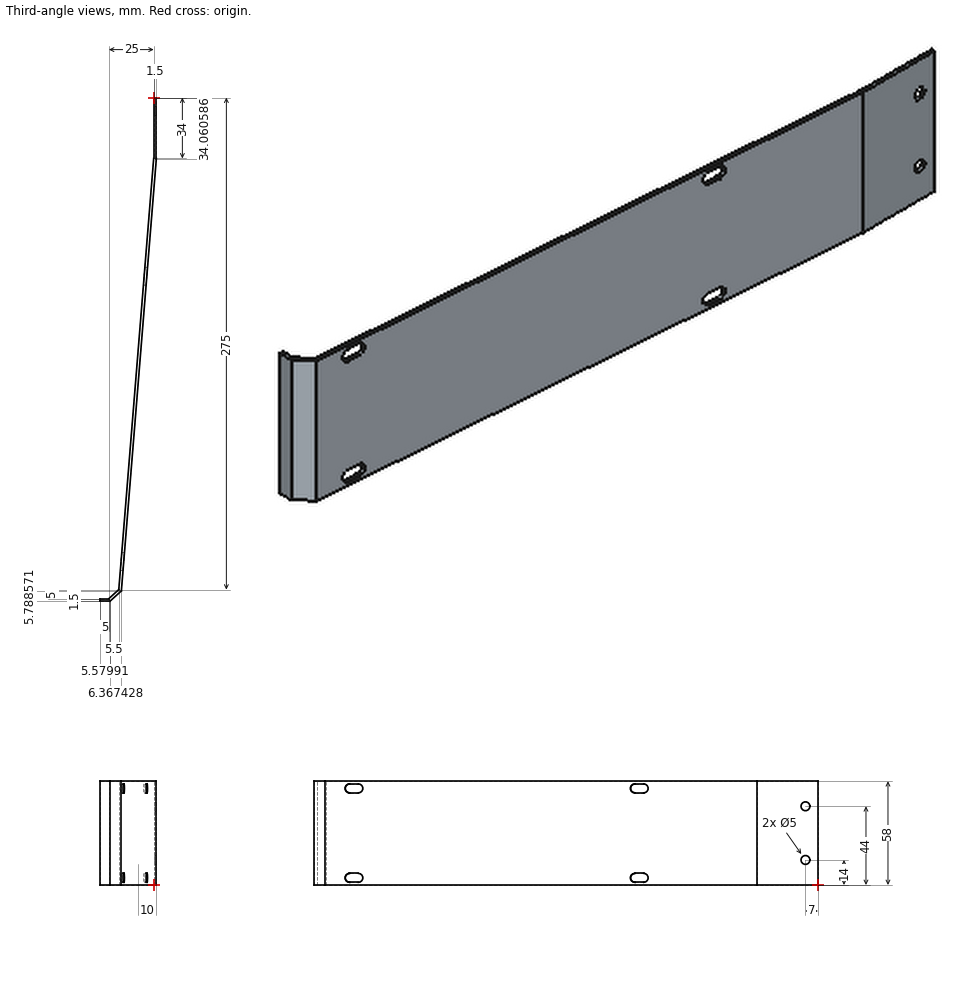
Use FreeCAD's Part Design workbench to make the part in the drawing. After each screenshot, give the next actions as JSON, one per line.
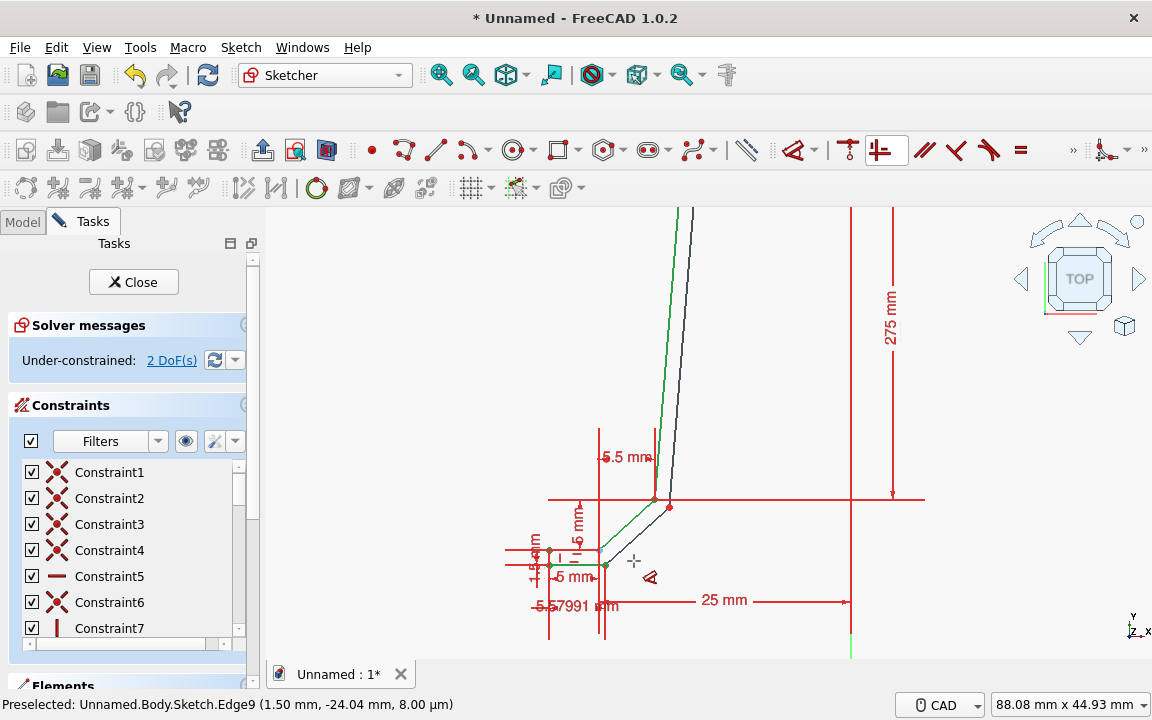
{"action": "left_click", "coordinate": [624, 548]}
{"action": "left_click", "coordinate": [652, 599]}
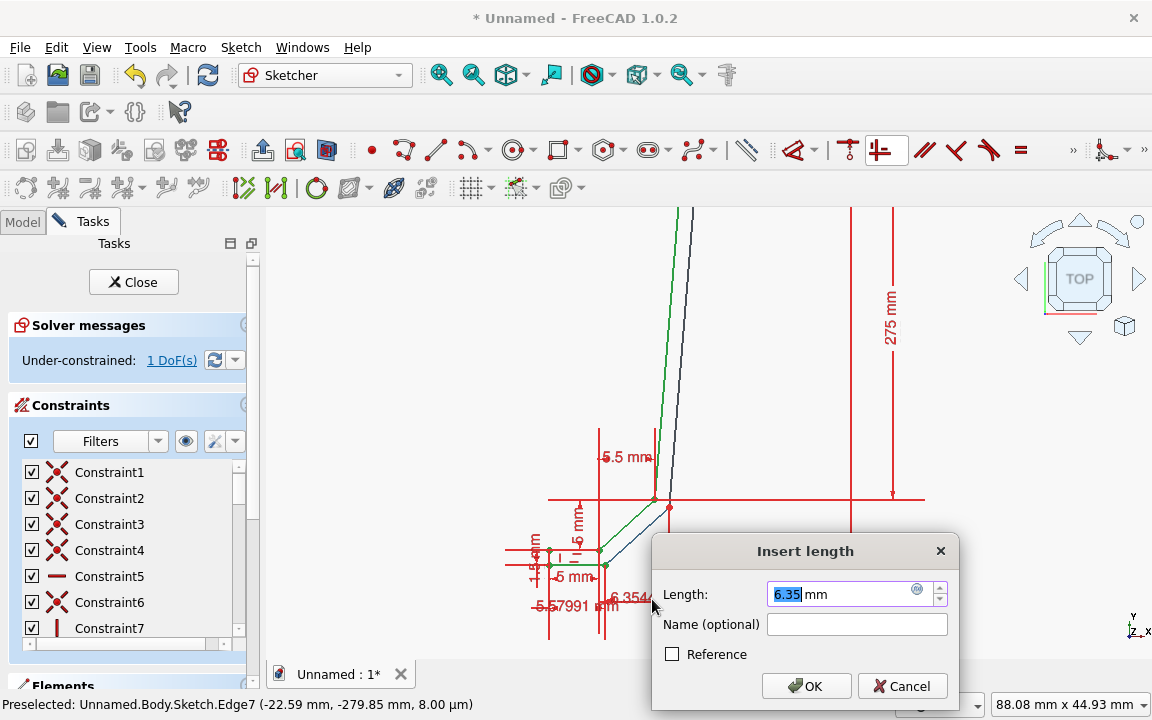
{"action": "type", "text": "6.367428"}
{"action": "key", "text": "Return"}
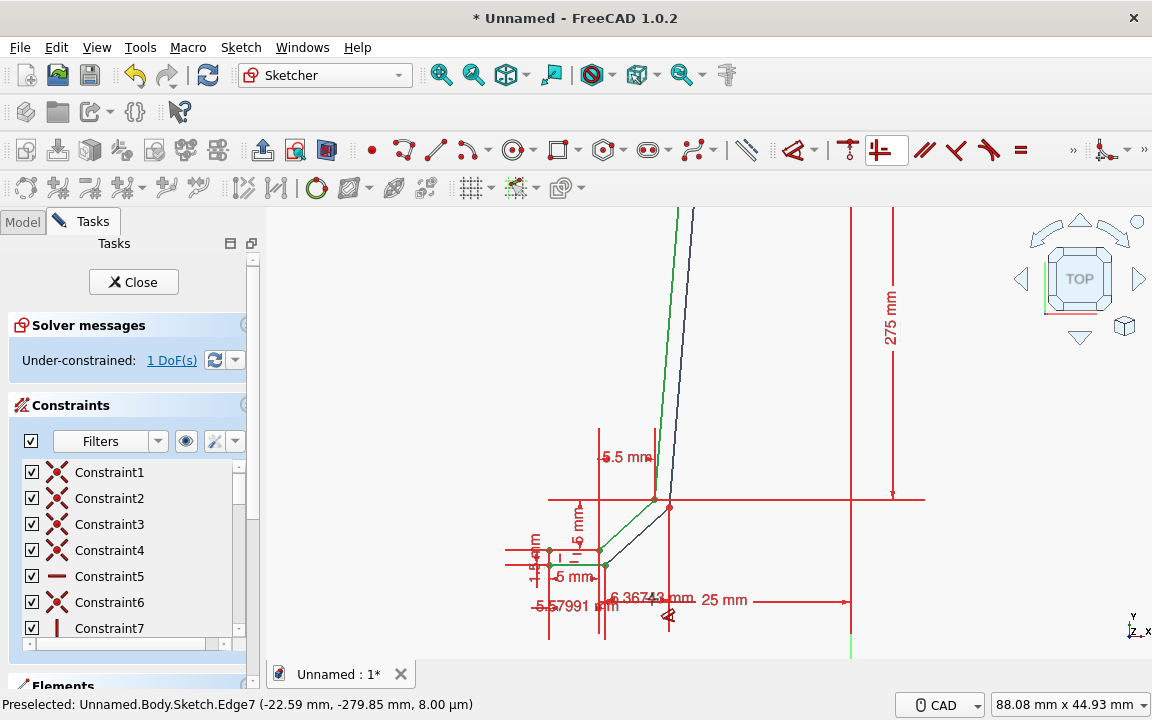
{"action": "left_click", "coordinate": [624, 548]}
{"action": "left_click", "coordinate": [703, 537]}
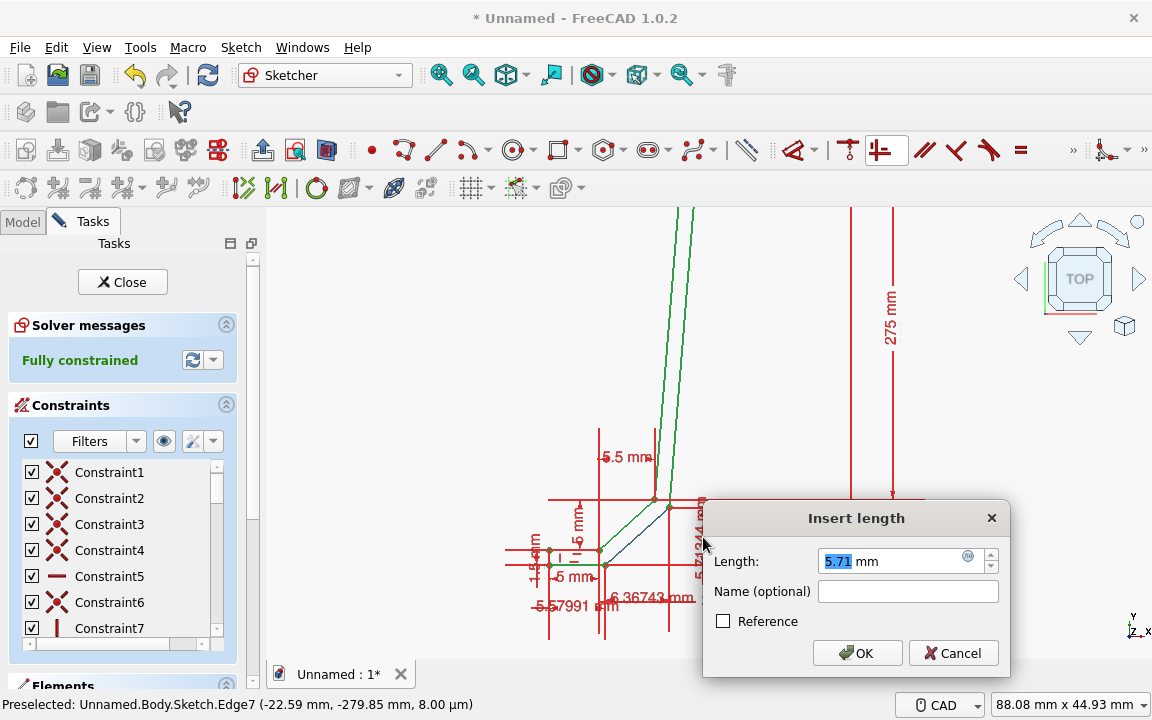
{"action": "type", "text": "5.788571"}
{"action": "key", "text": "Return"}
{"action": "key", "text": "Escape"}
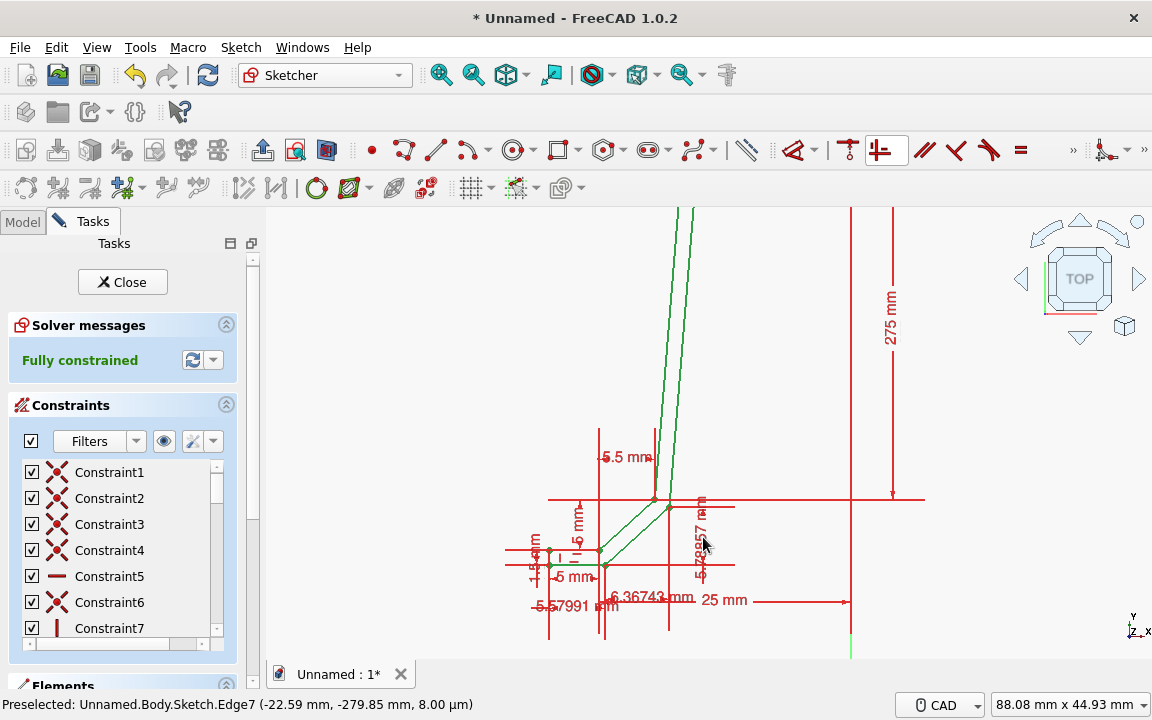
{"action": "left_click", "coordinate": [123, 282]}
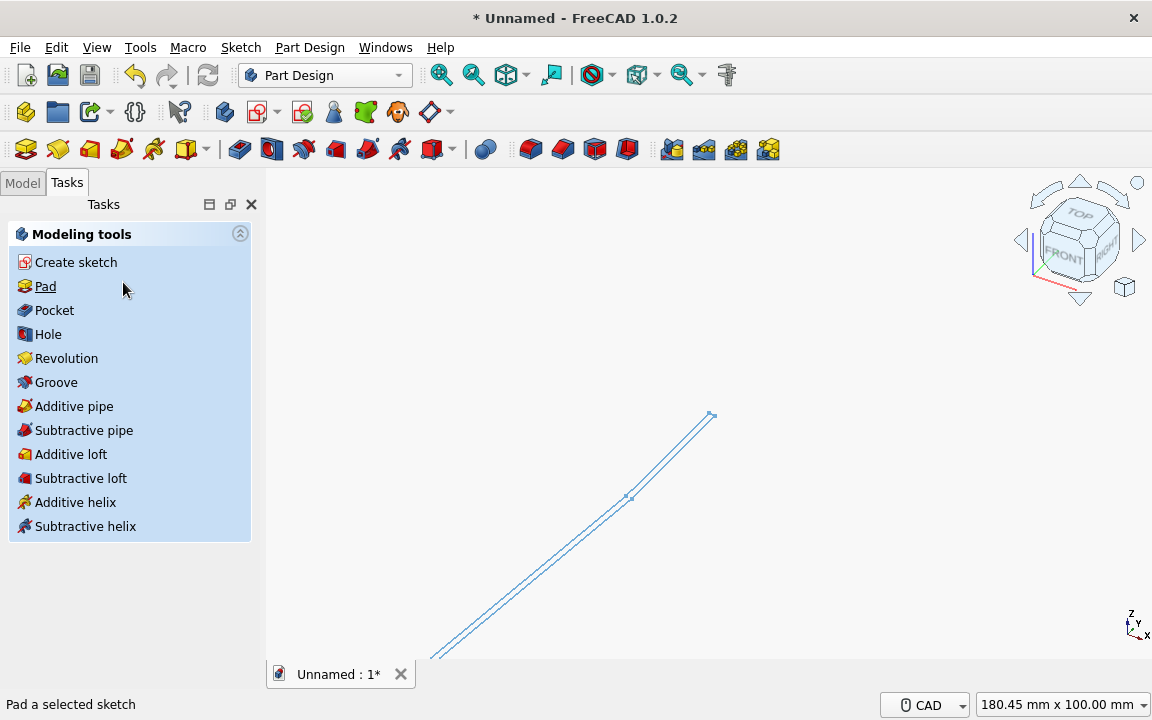
{"action": "left_click", "coordinate": [26, 150]}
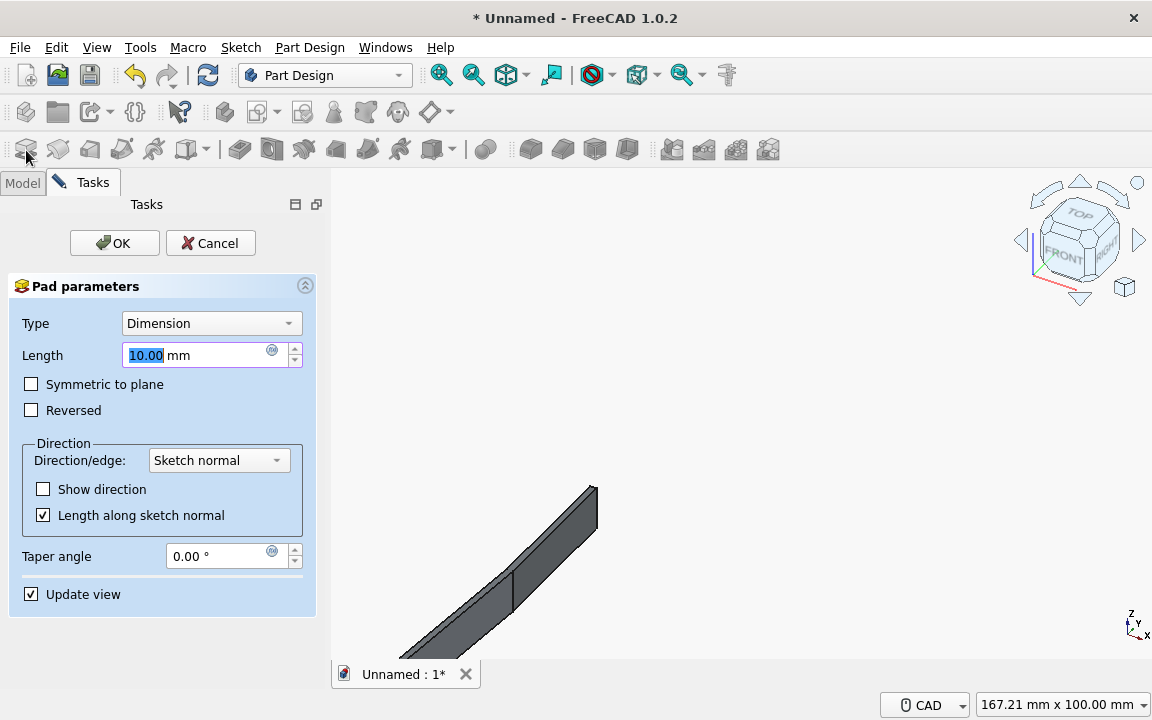
{"action": "type", "text": "58"}
{"action": "key", "text": "Tab"}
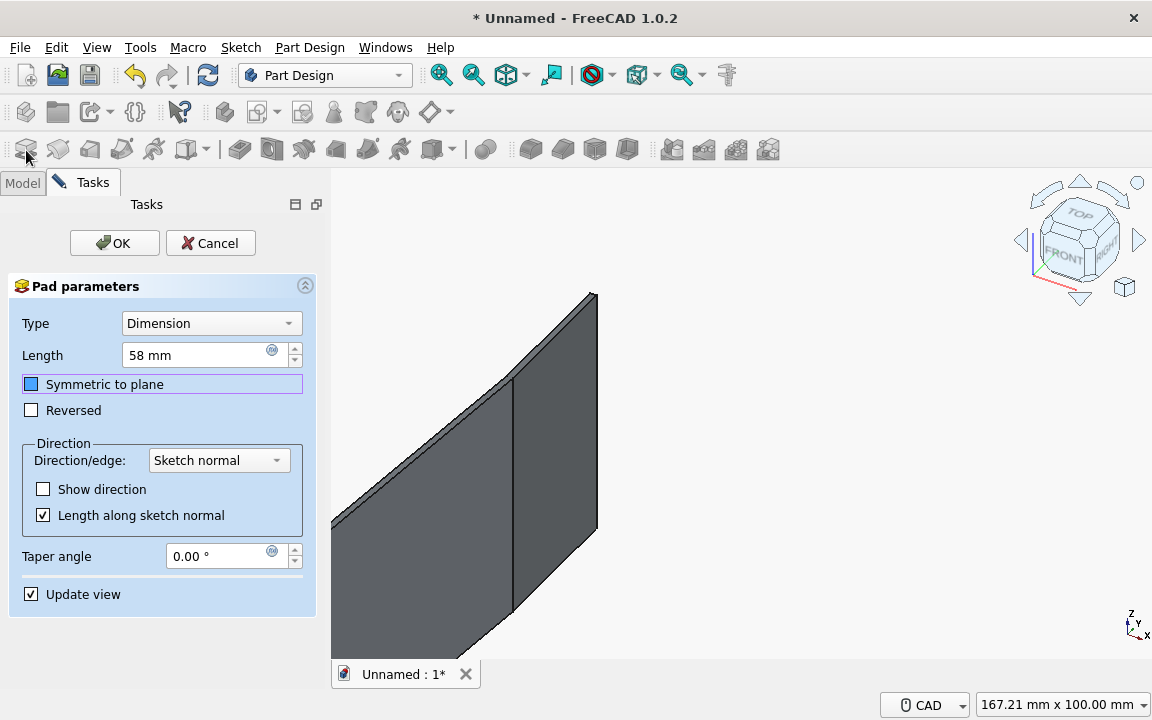
{"action": "left_click", "coordinate": [115, 243]}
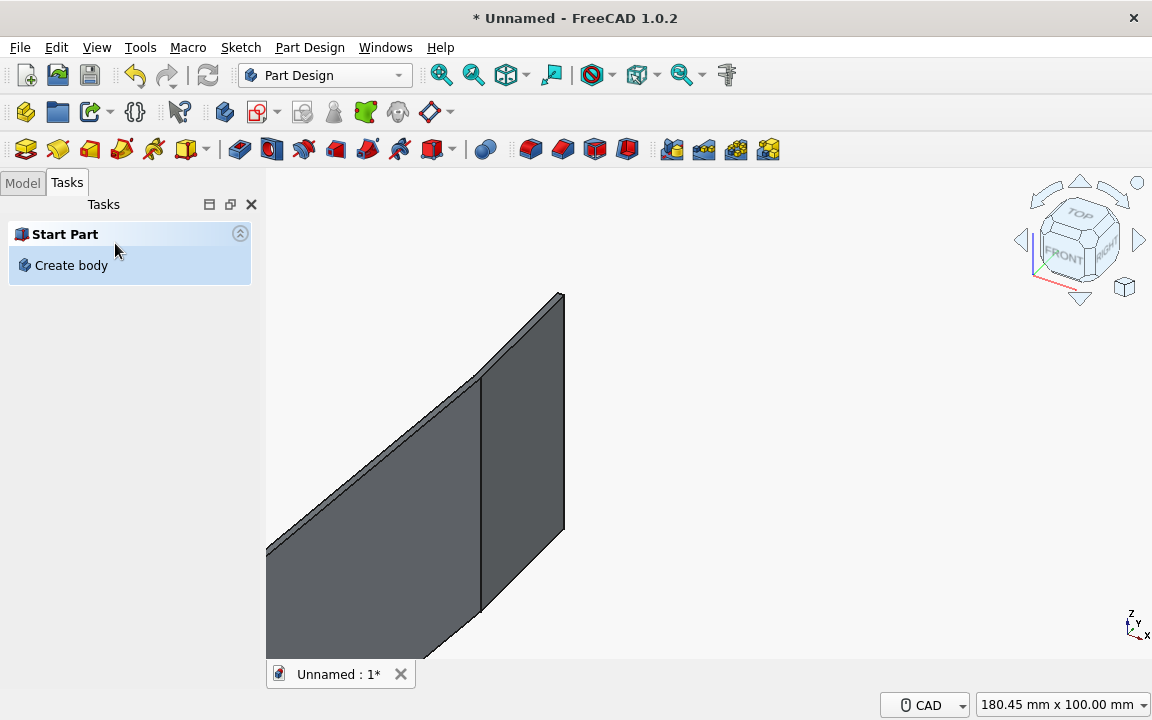
{"action": "left_click", "coordinate": [442, 76]}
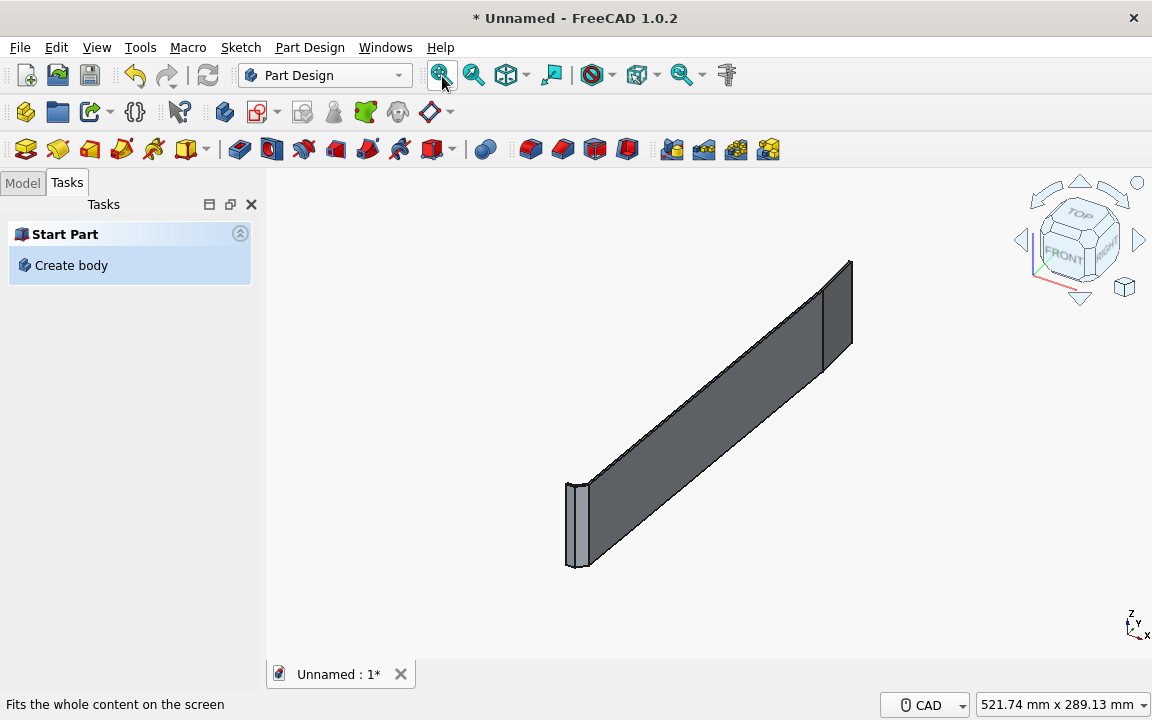
{"action": "left_click", "coordinate": [837, 304]}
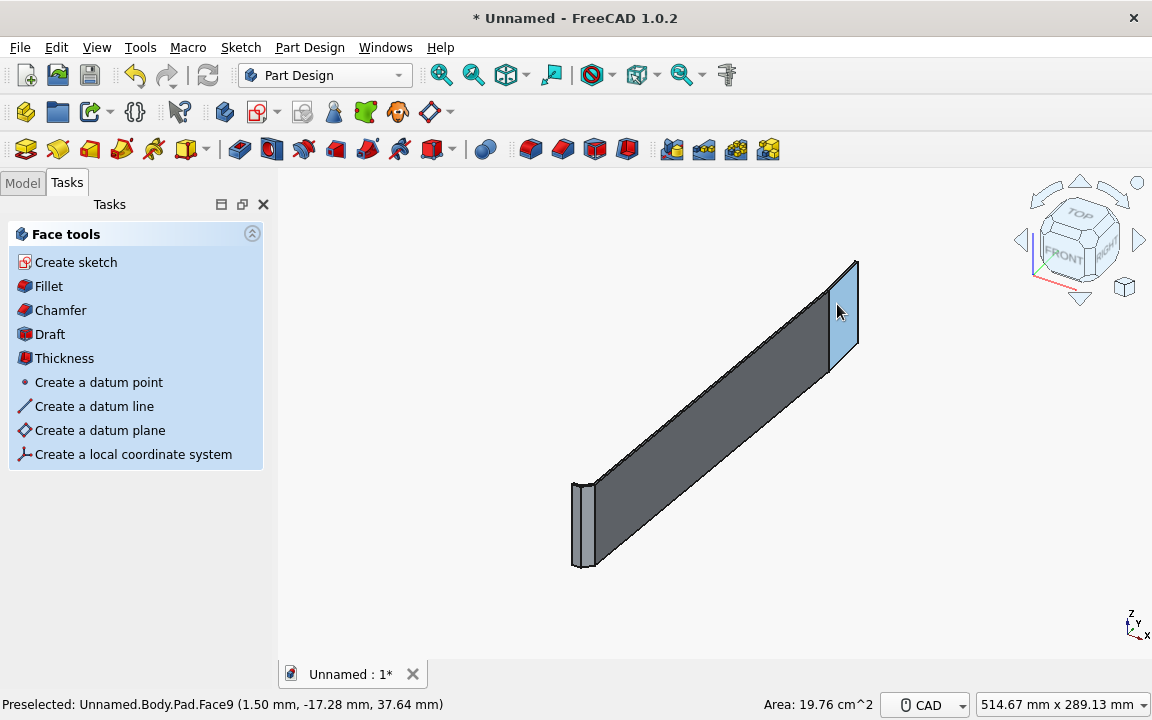
{"action": "left_click", "coordinate": [258, 112]}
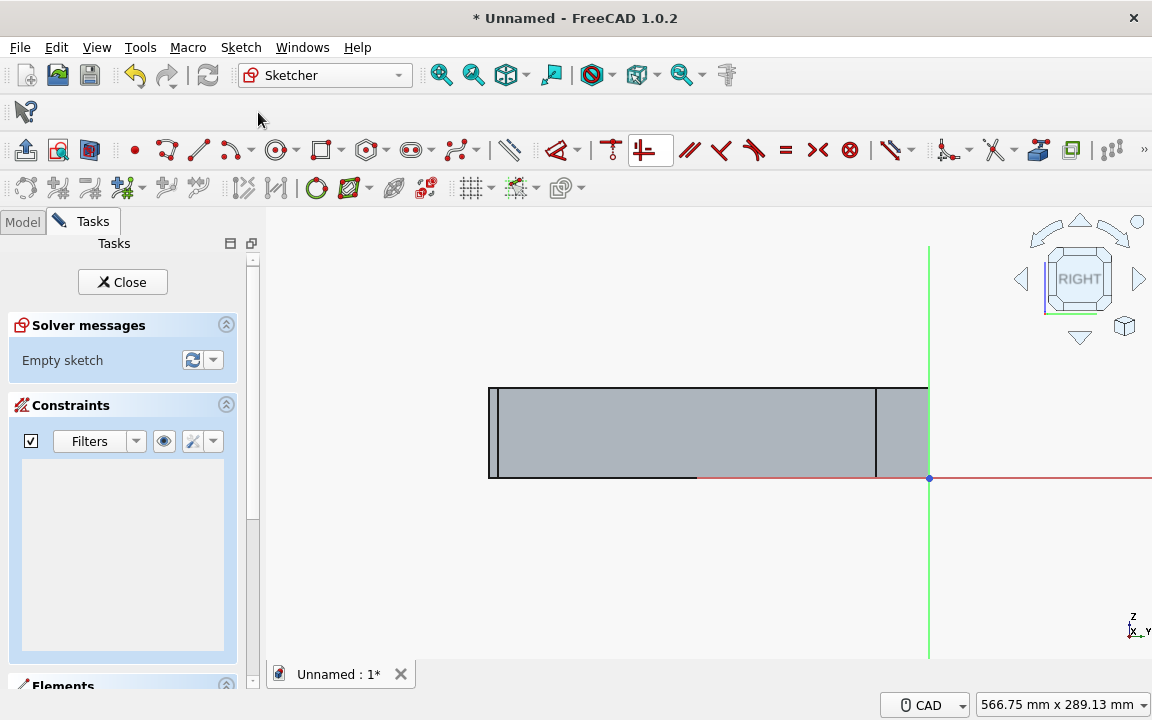
{"action": "scroll", "coordinate": [987, 445], "scroll_direction": "up", "scroll_amount": 7}